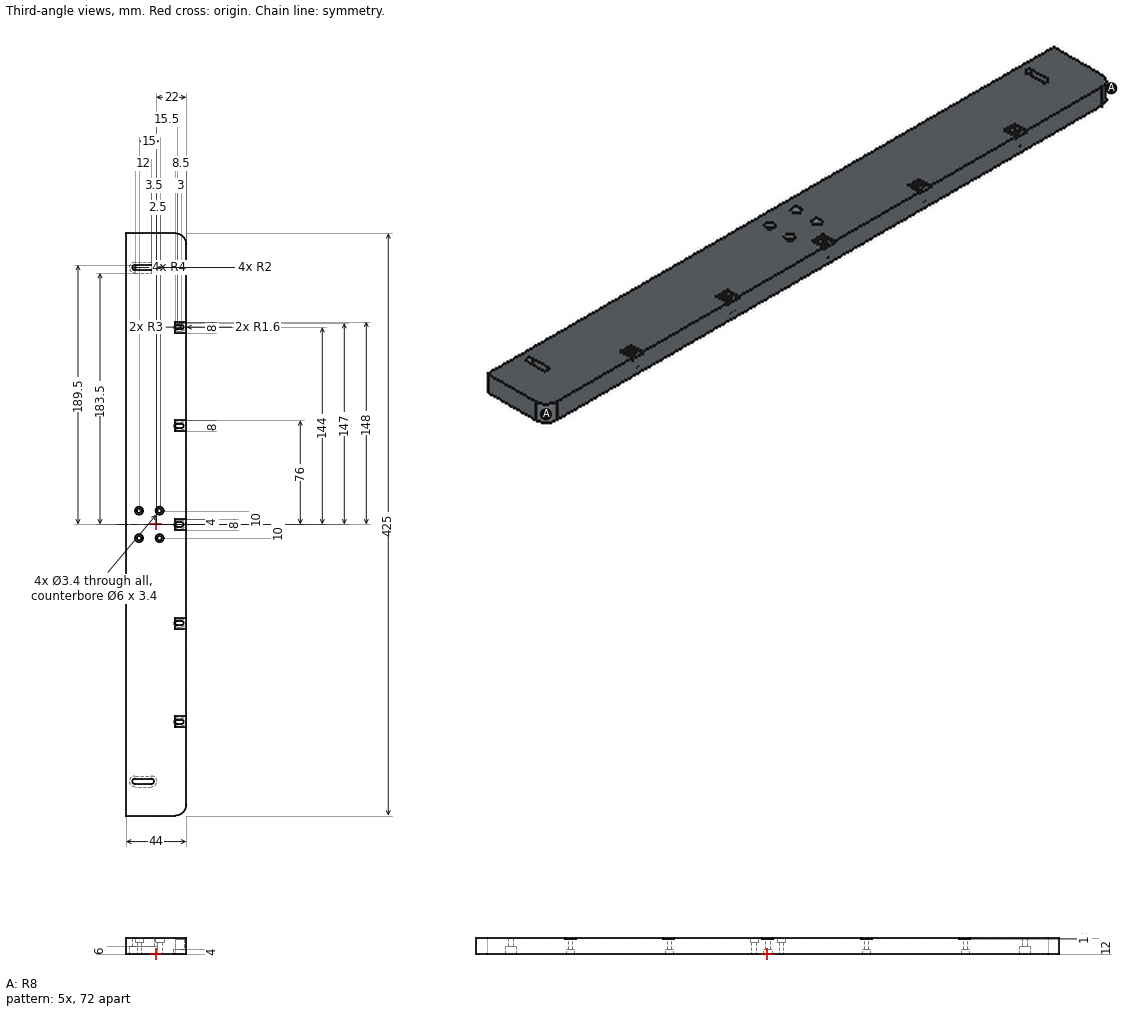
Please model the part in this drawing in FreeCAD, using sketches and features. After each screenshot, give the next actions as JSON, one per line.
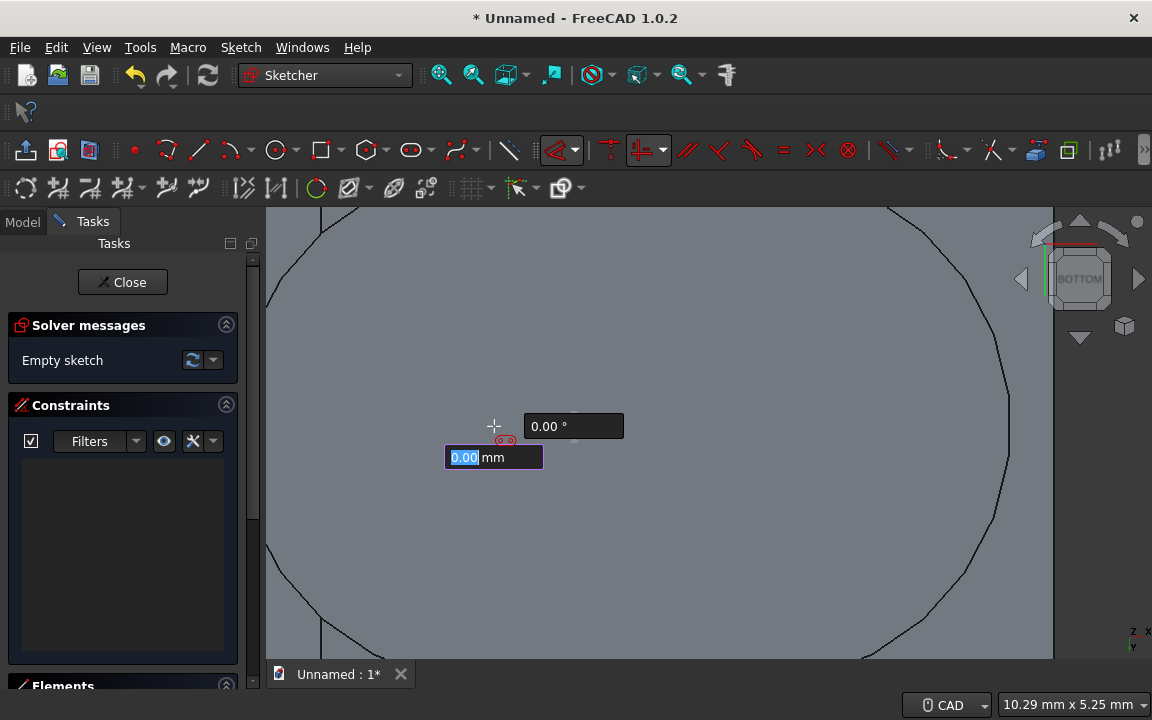
{"action": "left_click", "coordinate": [752, 426]}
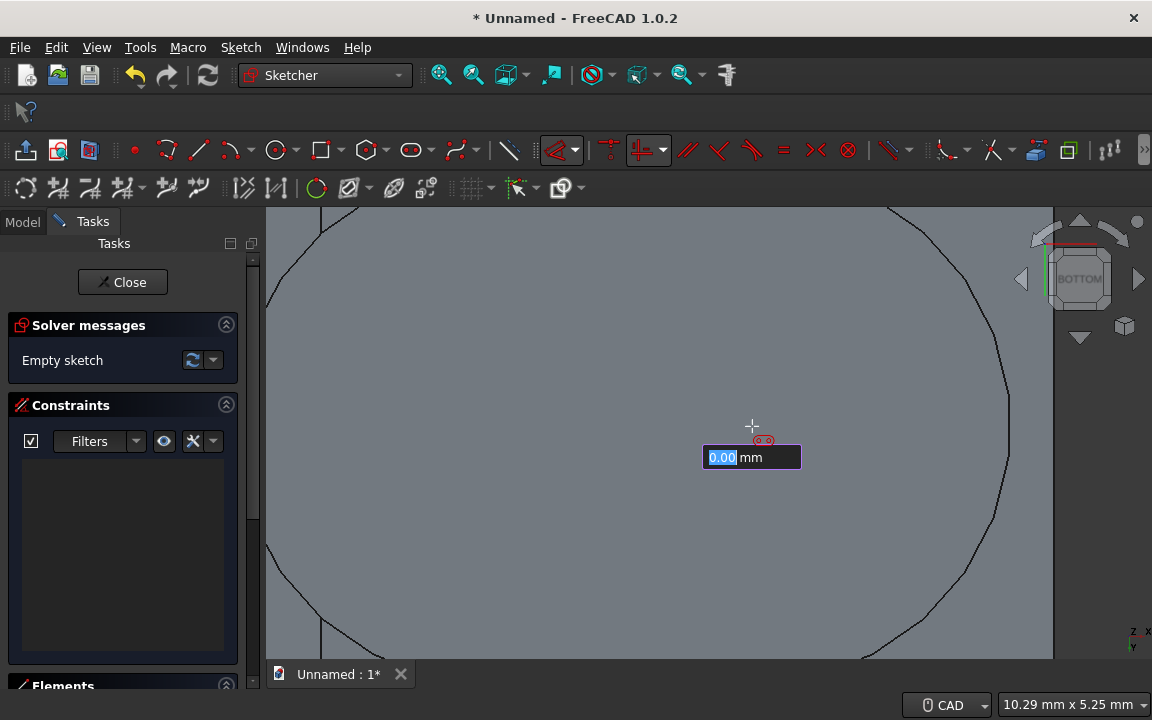
{"action": "left_click", "coordinate": [623, 564]}
{"action": "key", "text": "Escape"}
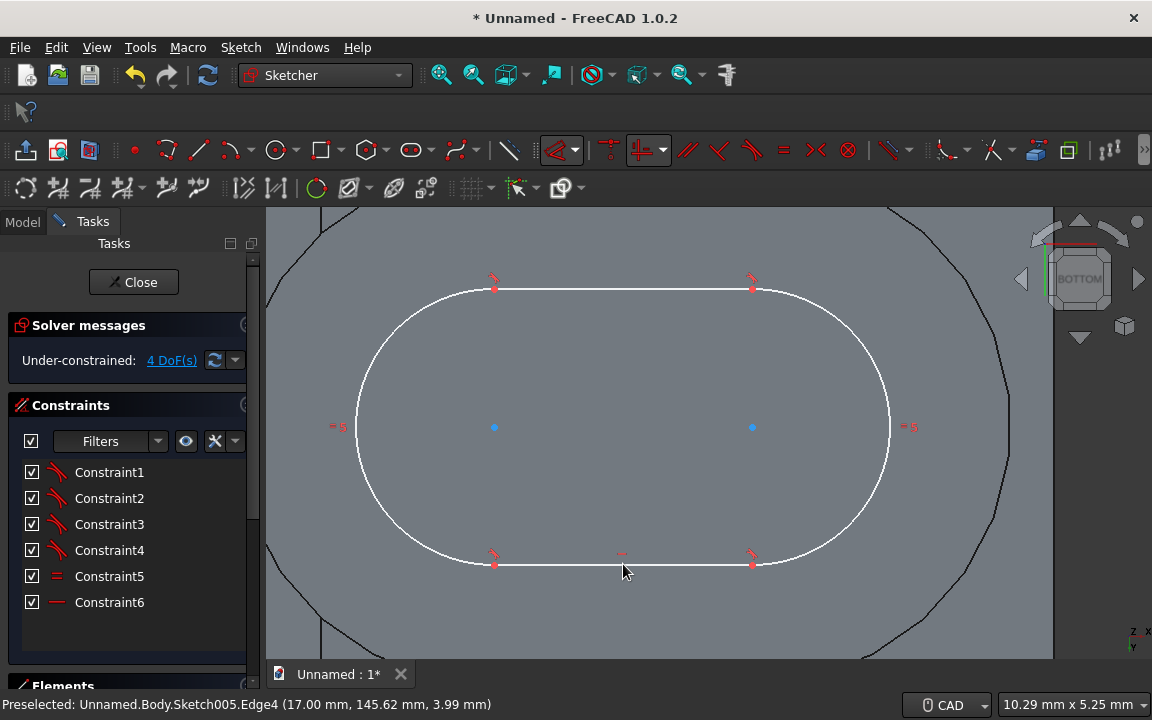
{"action": "left_click", "coordinate": [382, 346]}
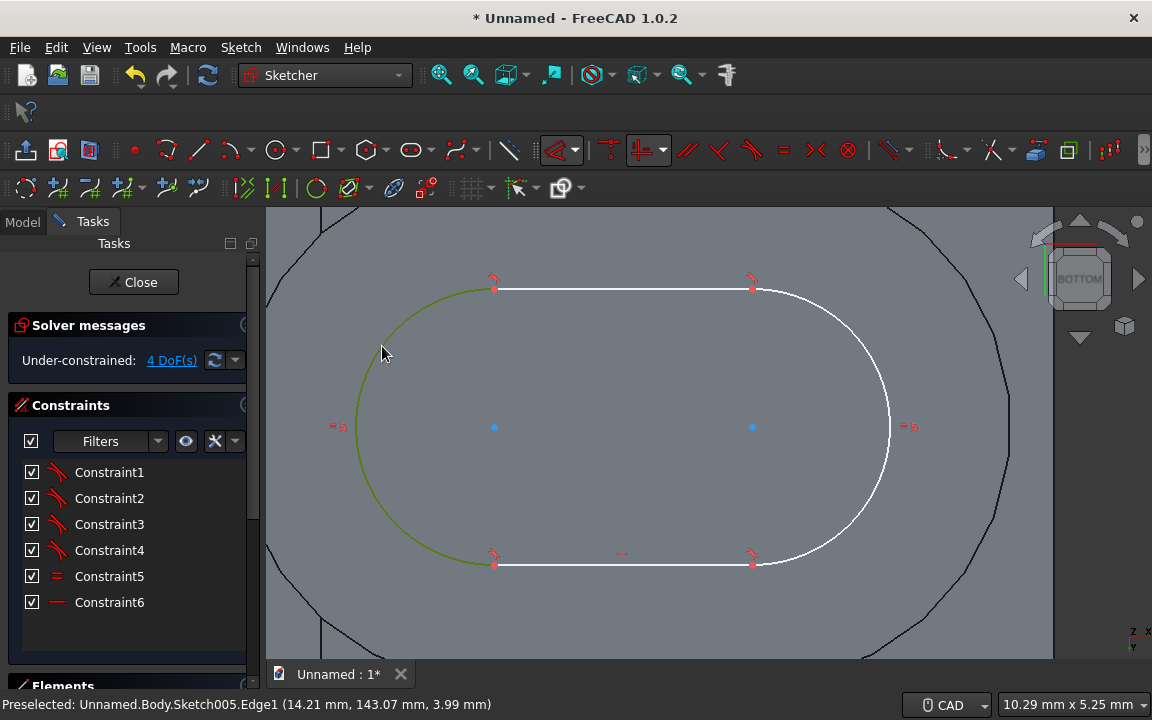
{"action": "key", "text": "k r"}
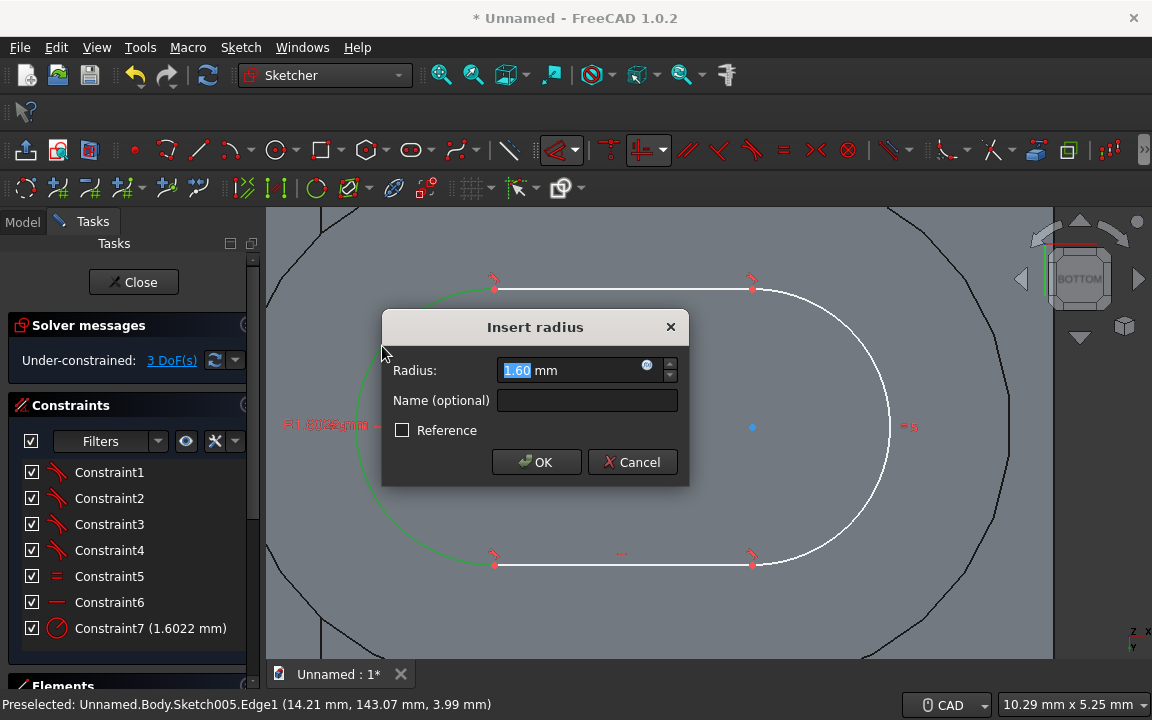
{"action": "type", "text": "1.6"}
{"action": "key", "text": "Return"}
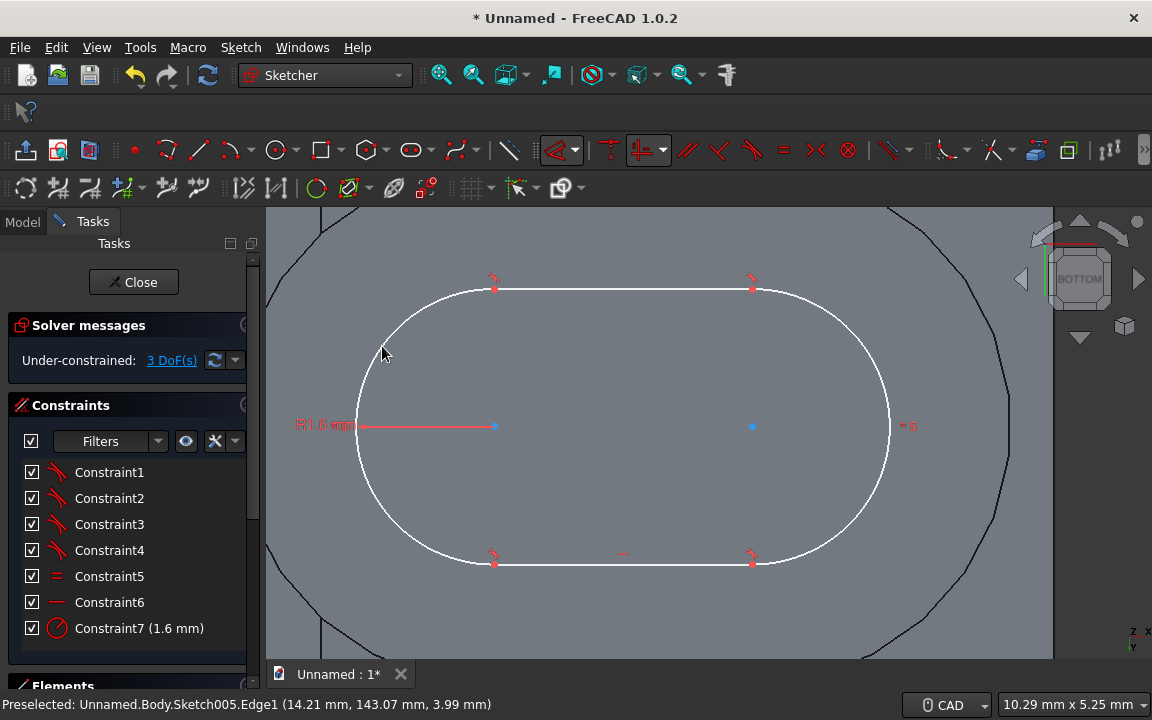
{"action": "left_click", "coordinate": [571, 289]}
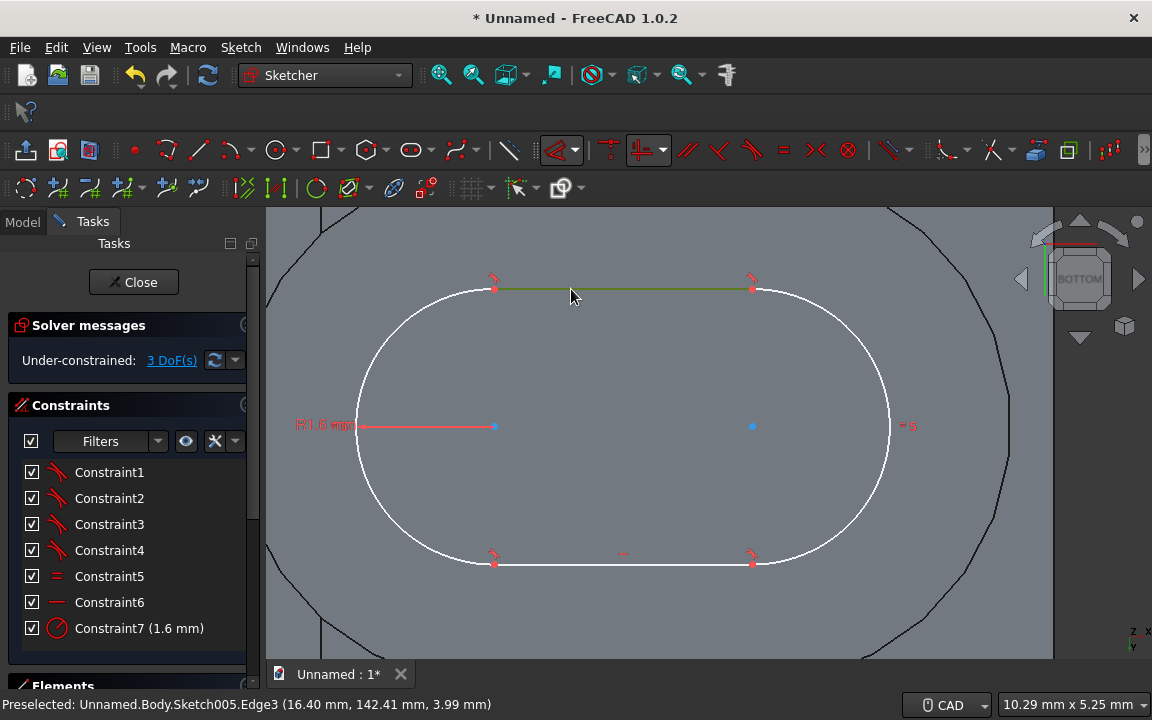
{"action": "key", "text": "l"}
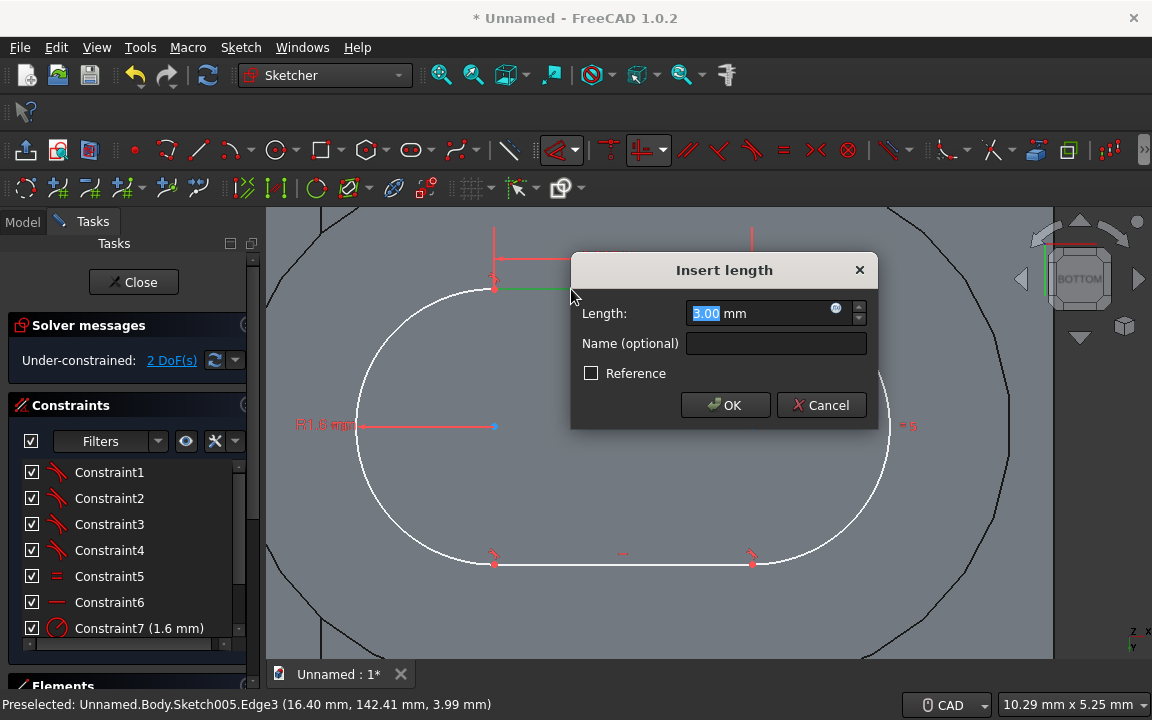
{"action": "type", "text": "3"}
{"action": "key", "text": "Return"}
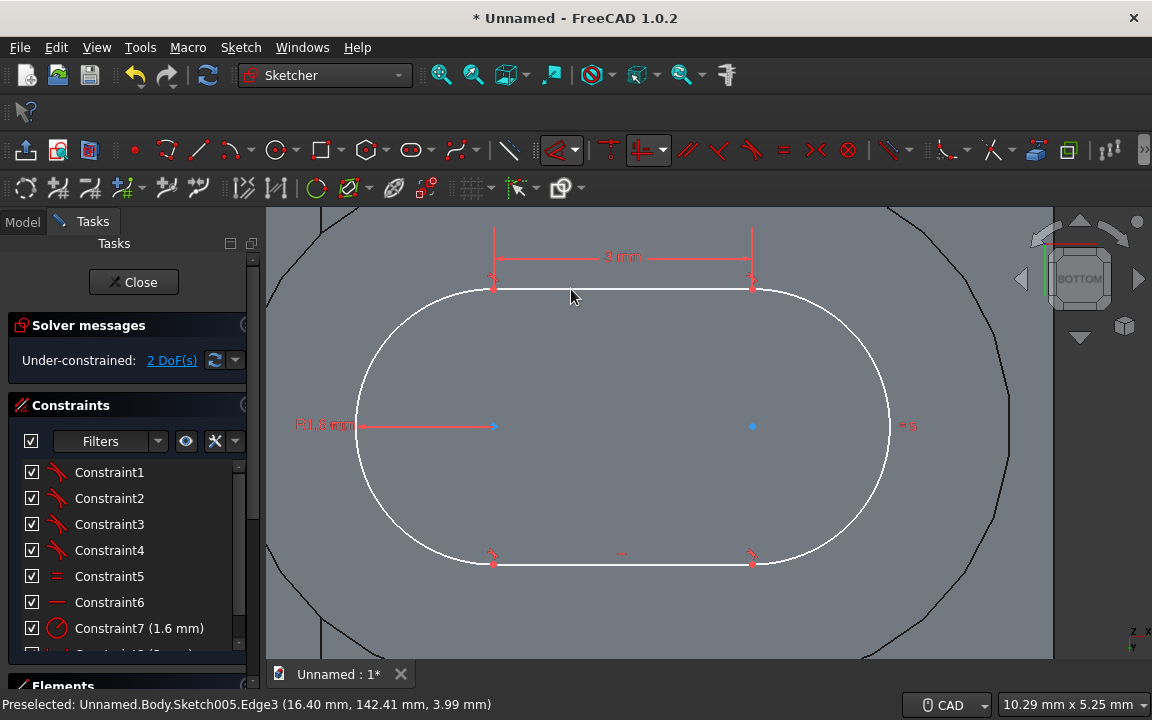
{"action": "left_click", "coordinate": [494, 427]}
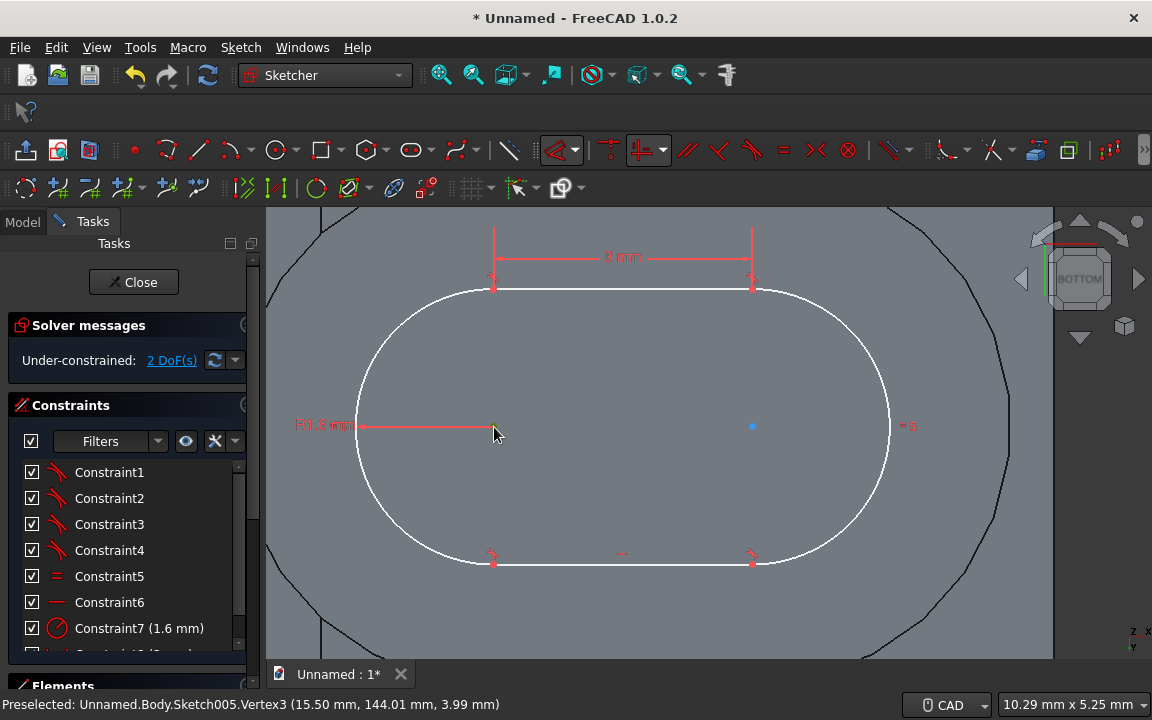
{"action": "left_click", "coordinate": [578, 150]}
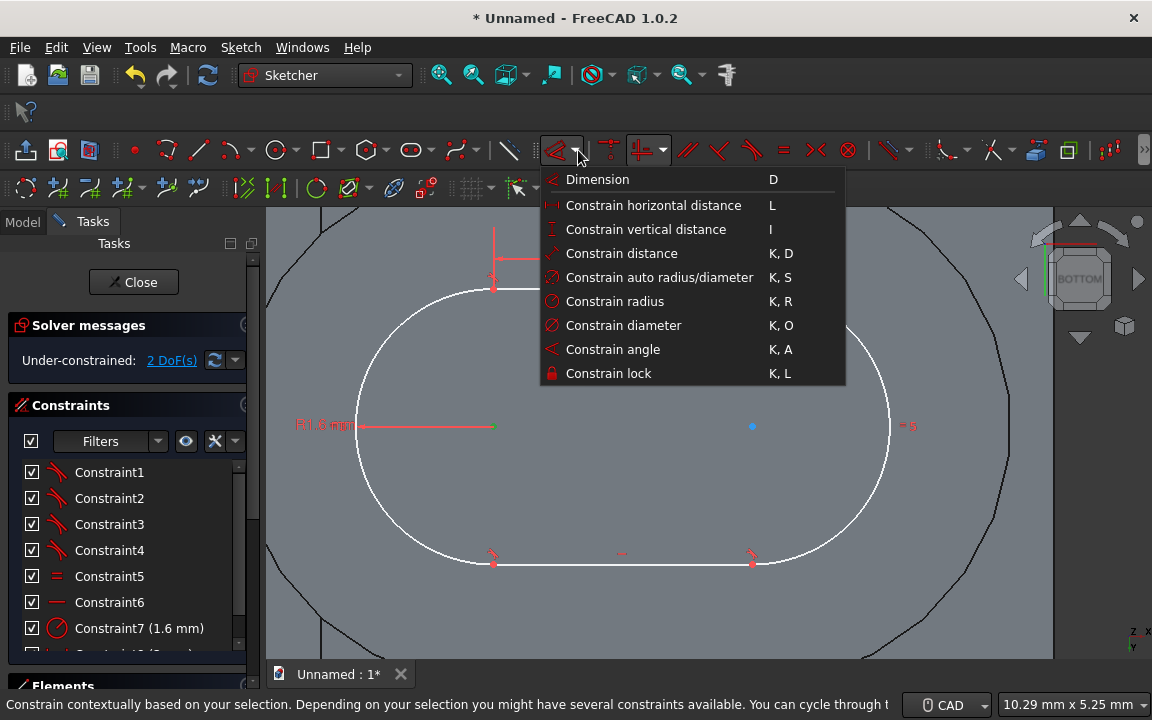
{"action": "left_click", "coordinate": [693, 229]}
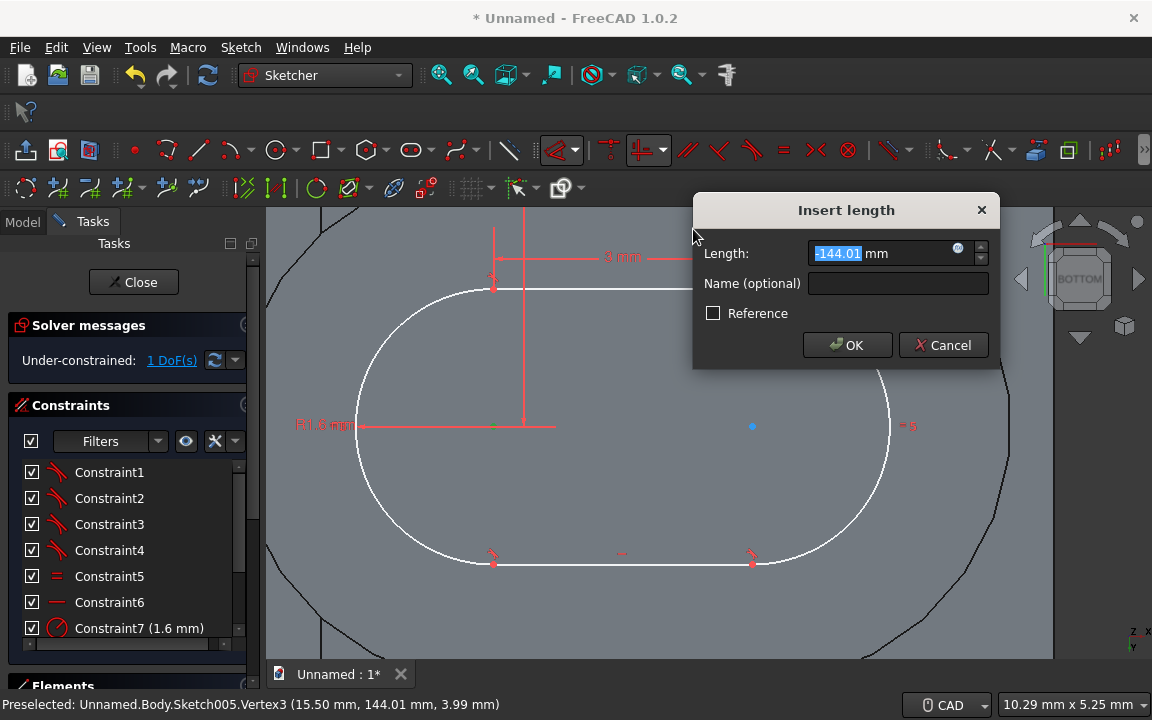
{"action": "type", "text": "-144"}
{"action": "key", "text": "Return"}